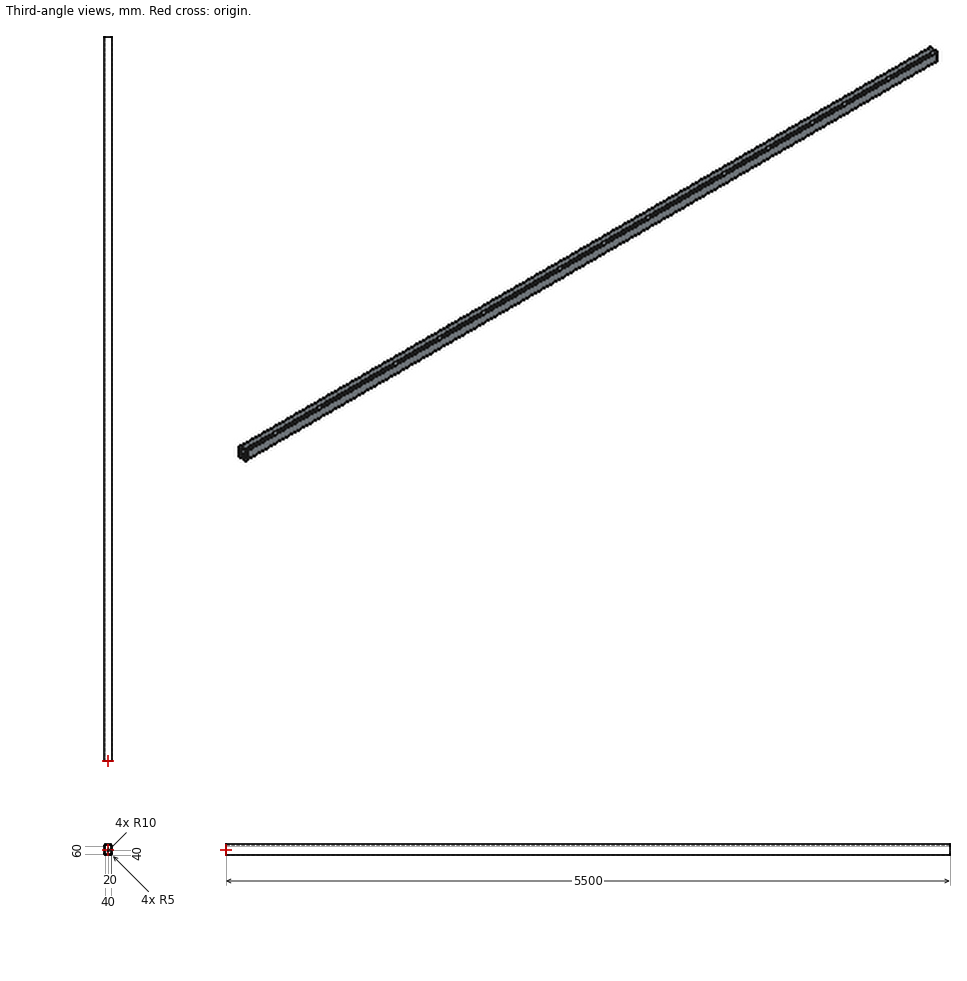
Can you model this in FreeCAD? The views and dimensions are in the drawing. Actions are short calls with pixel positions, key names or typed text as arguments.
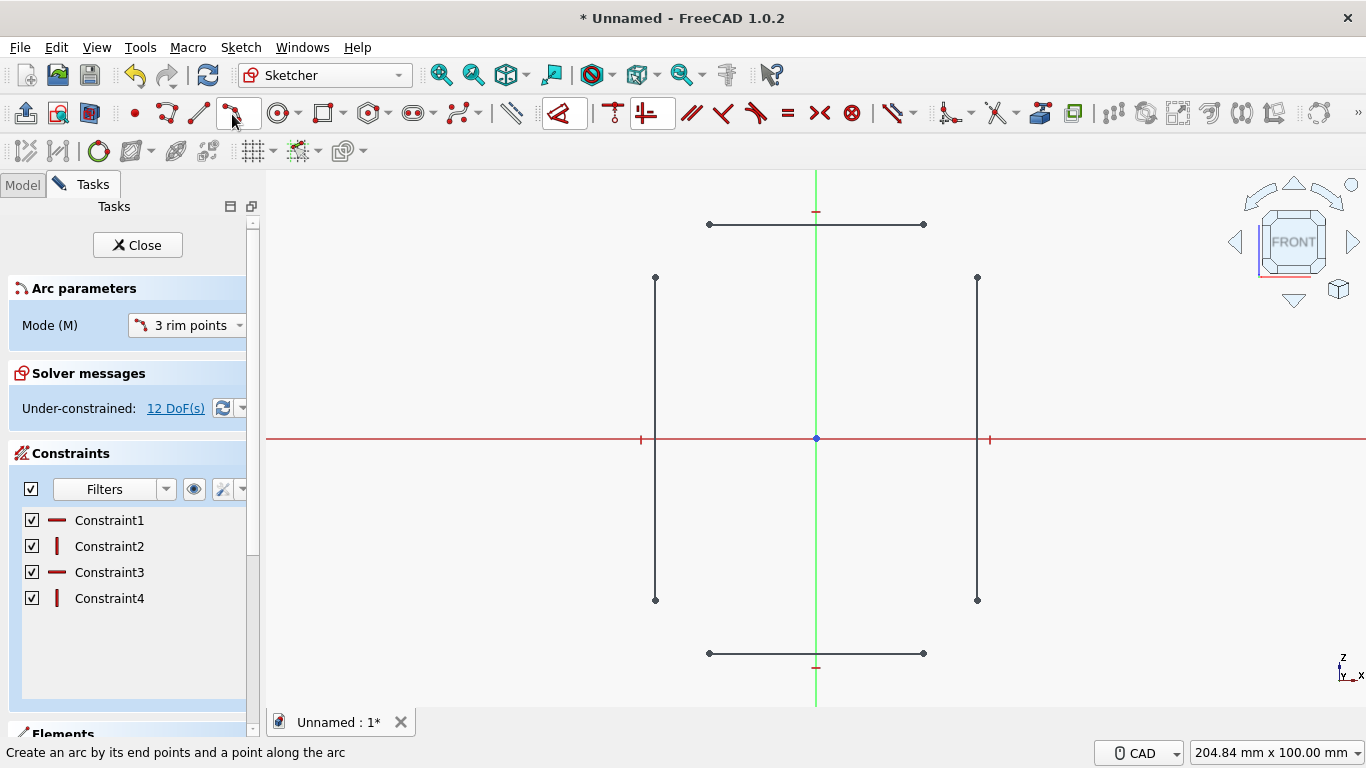
click(709, 654)
click(655, 601)
click(671, 638)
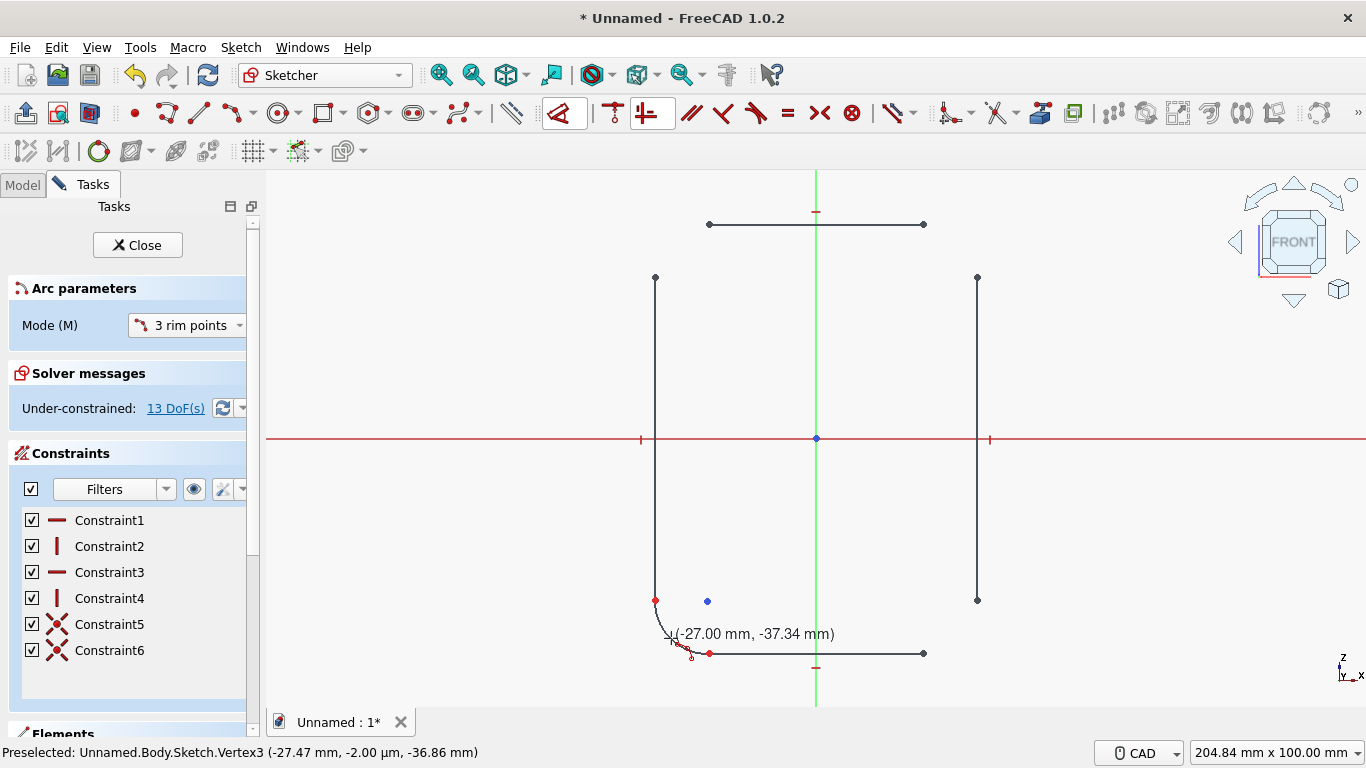
click(655, 278)
click(709, 225)
click(671, 239)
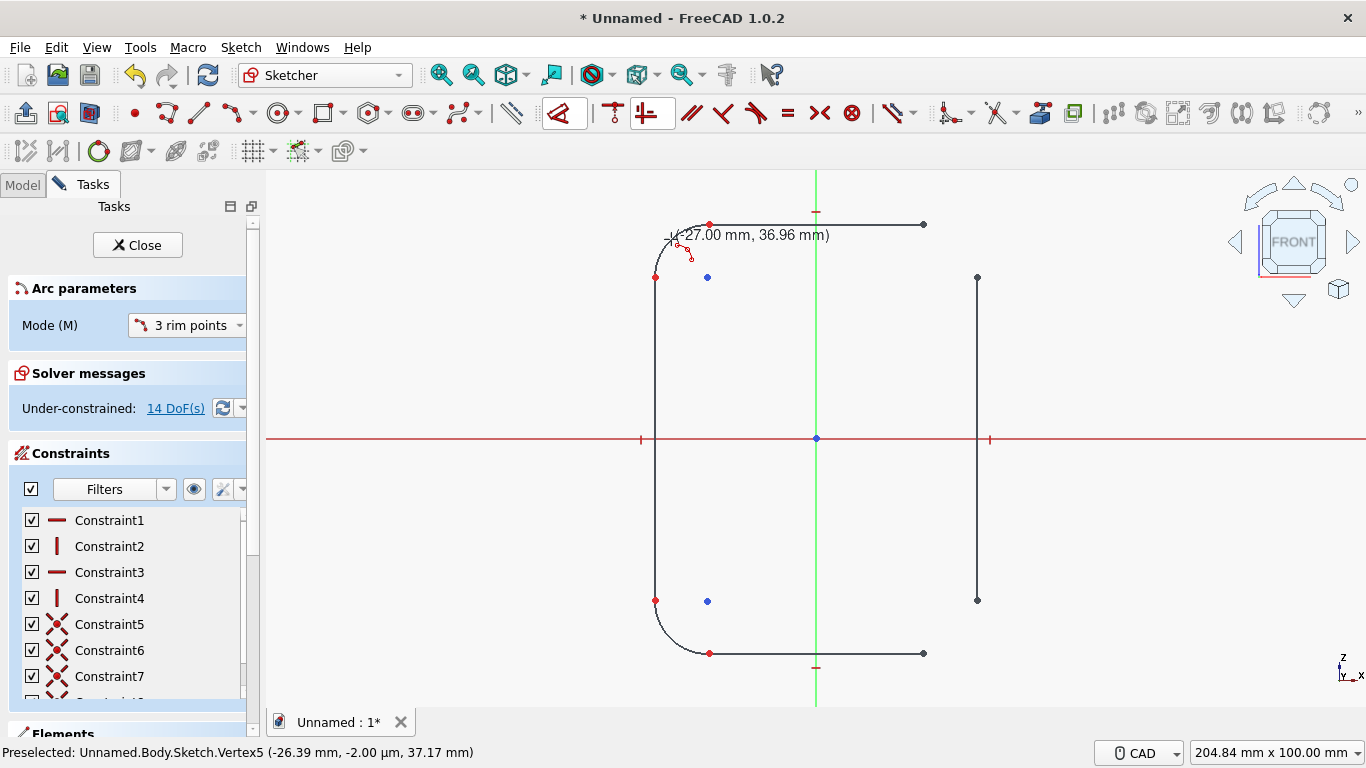
click(923, 225)
click(977, 278)
click(961, 239)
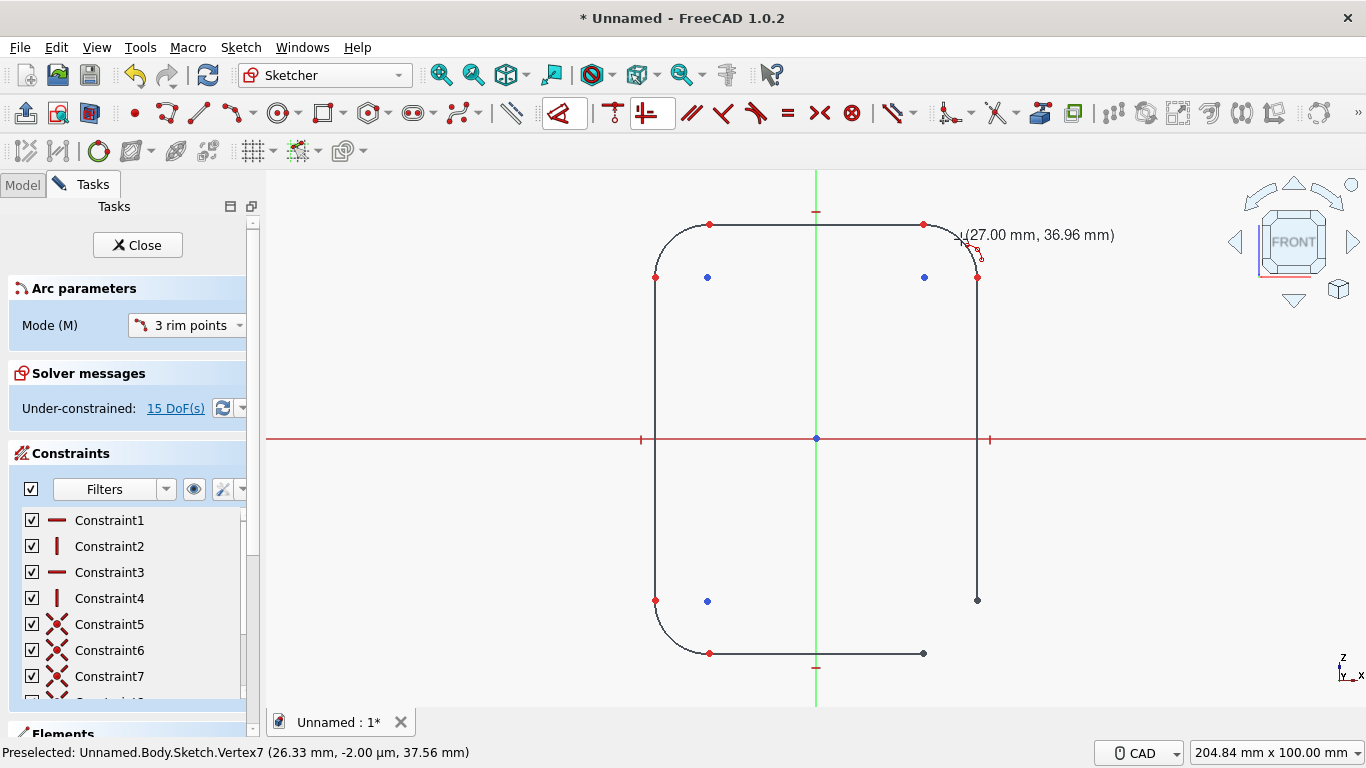
click(977, 601)
click(923, 654)
click(961, 638)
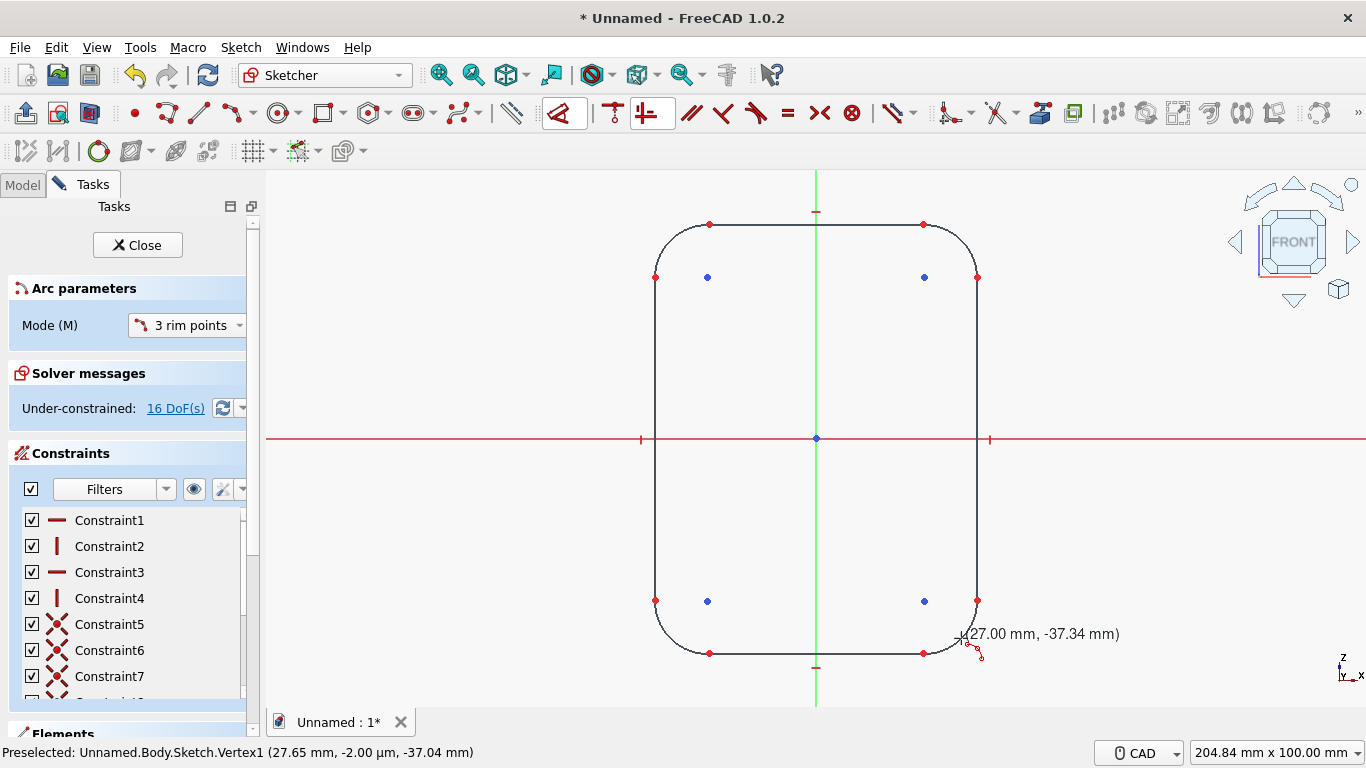
click(200, 114)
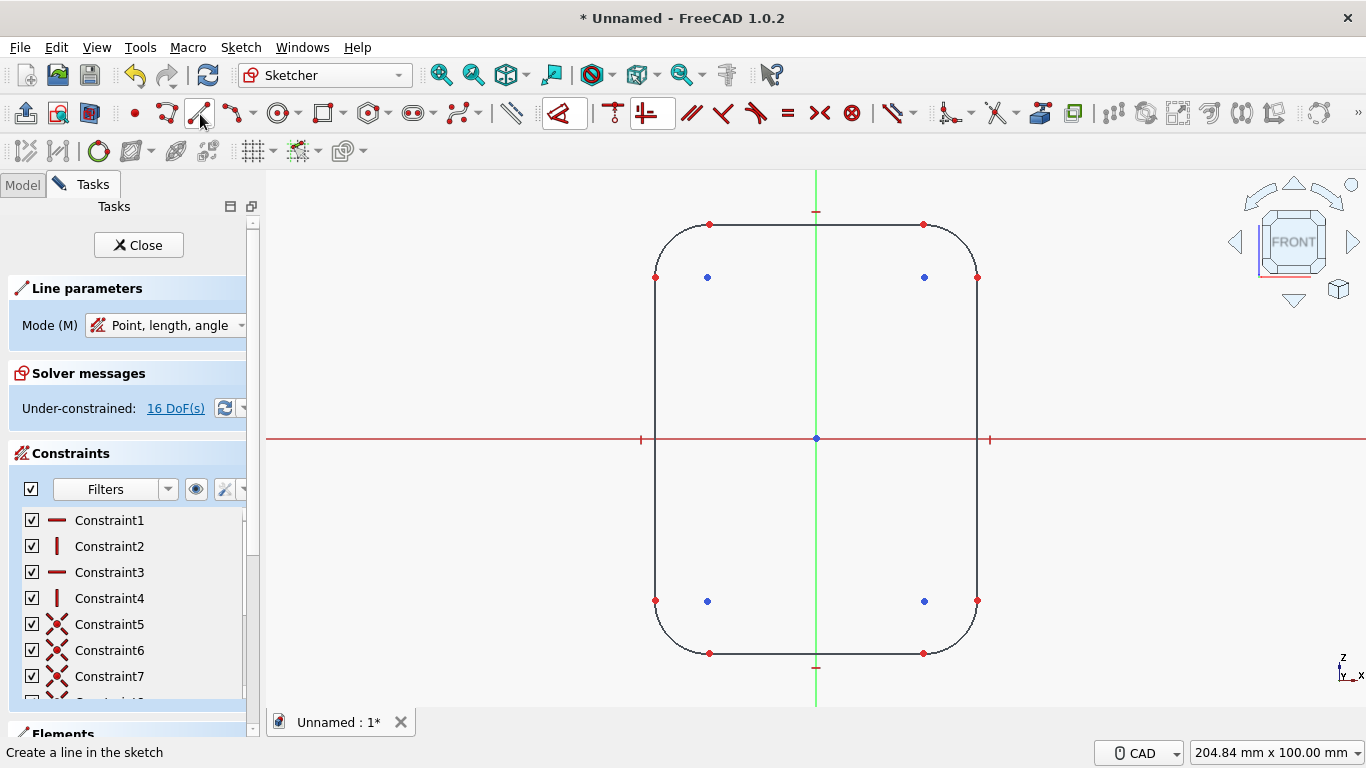
click(709, 626)
click(923, 626)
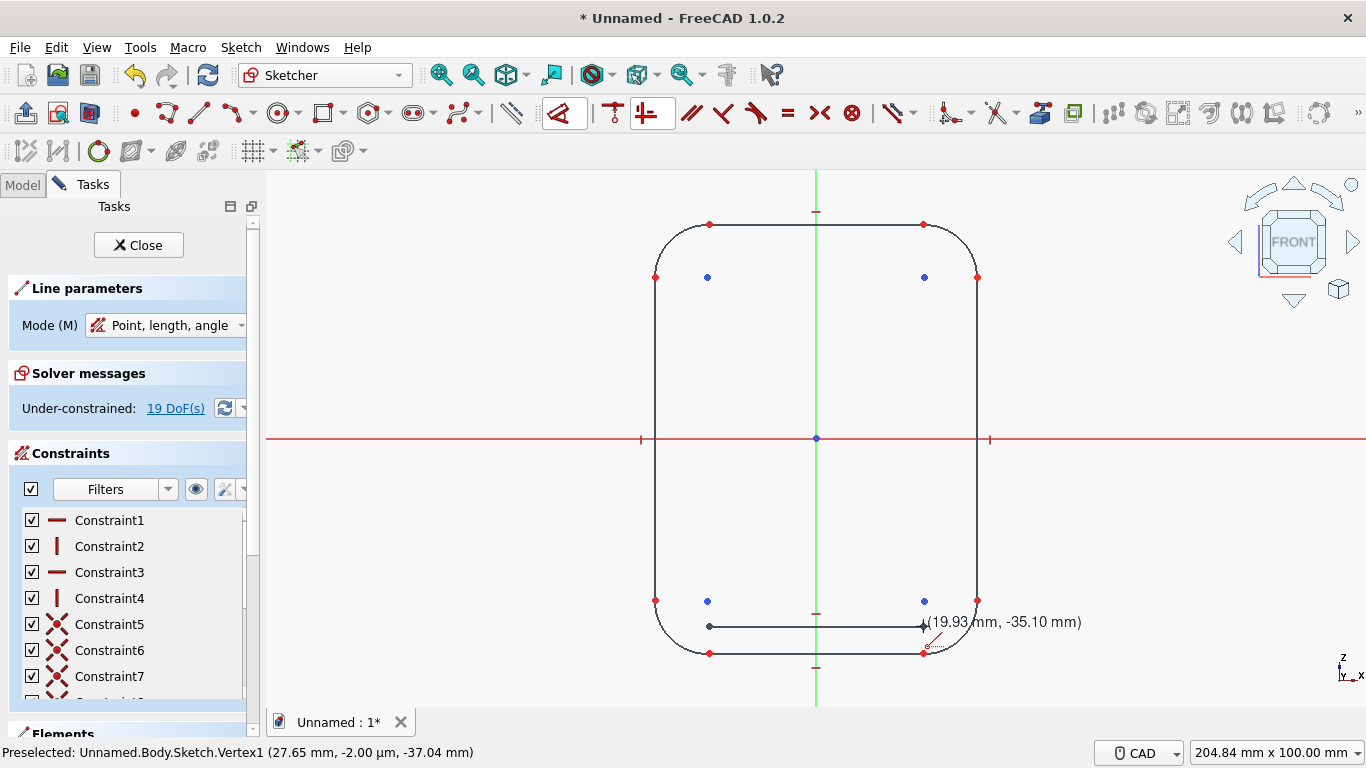
click(950, 600)
click(950, 277)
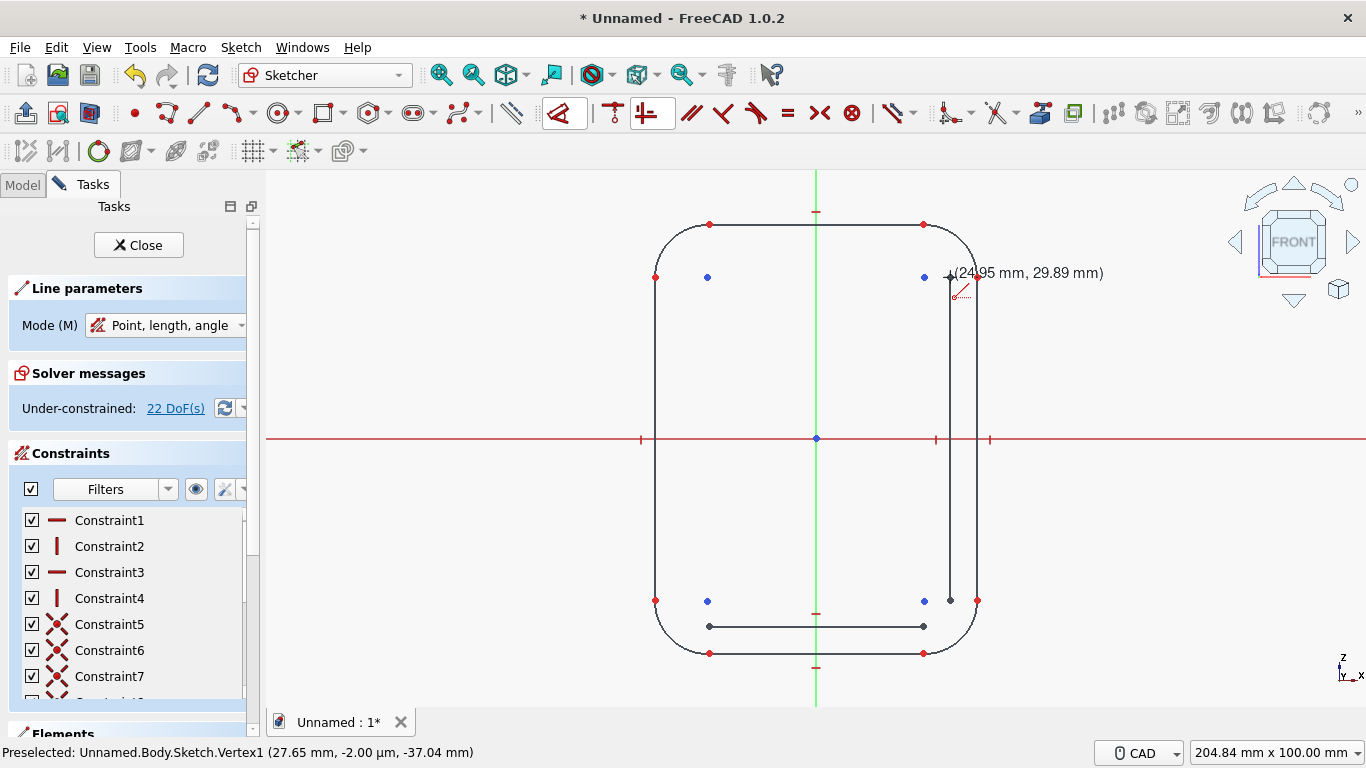
click(923, 251)
click(709, 251)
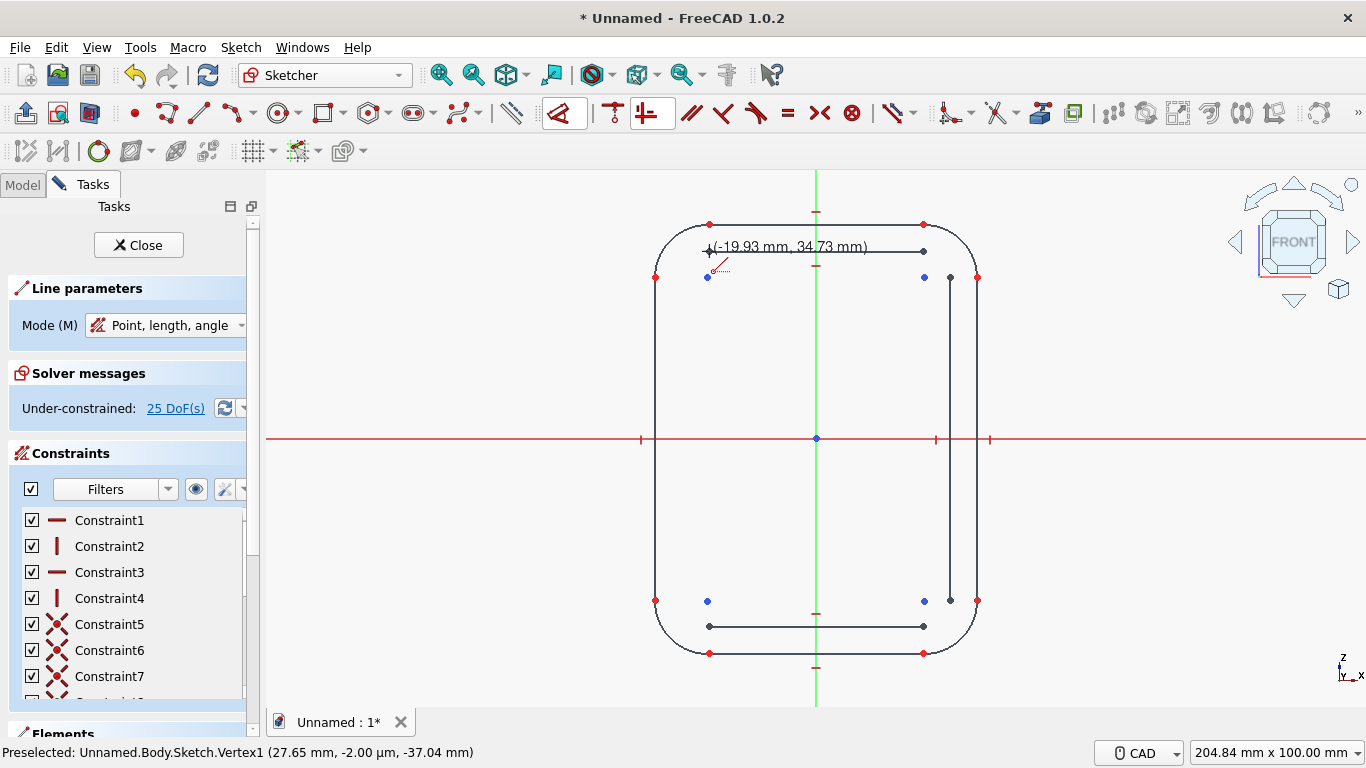
click(682, 277)
click(682, 600)